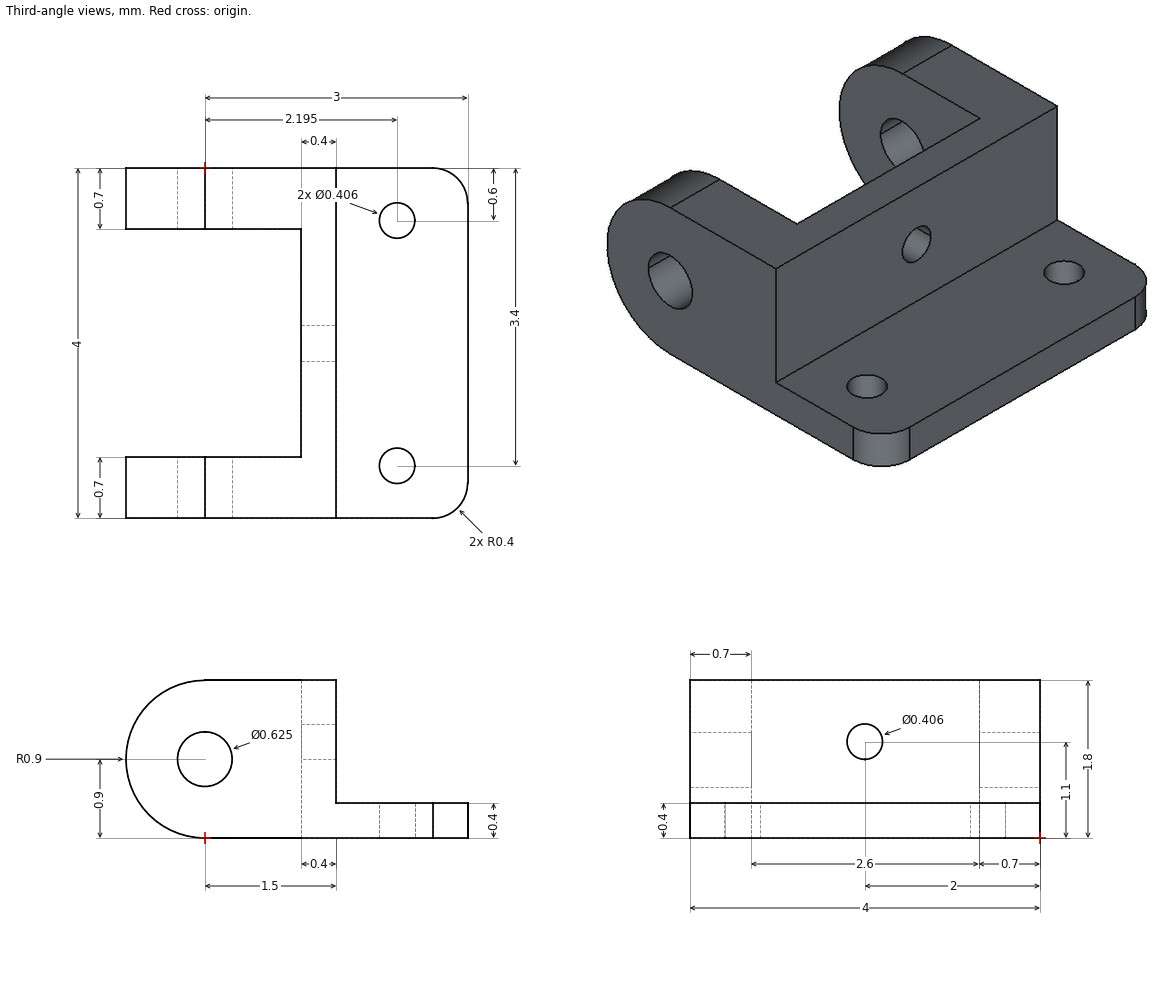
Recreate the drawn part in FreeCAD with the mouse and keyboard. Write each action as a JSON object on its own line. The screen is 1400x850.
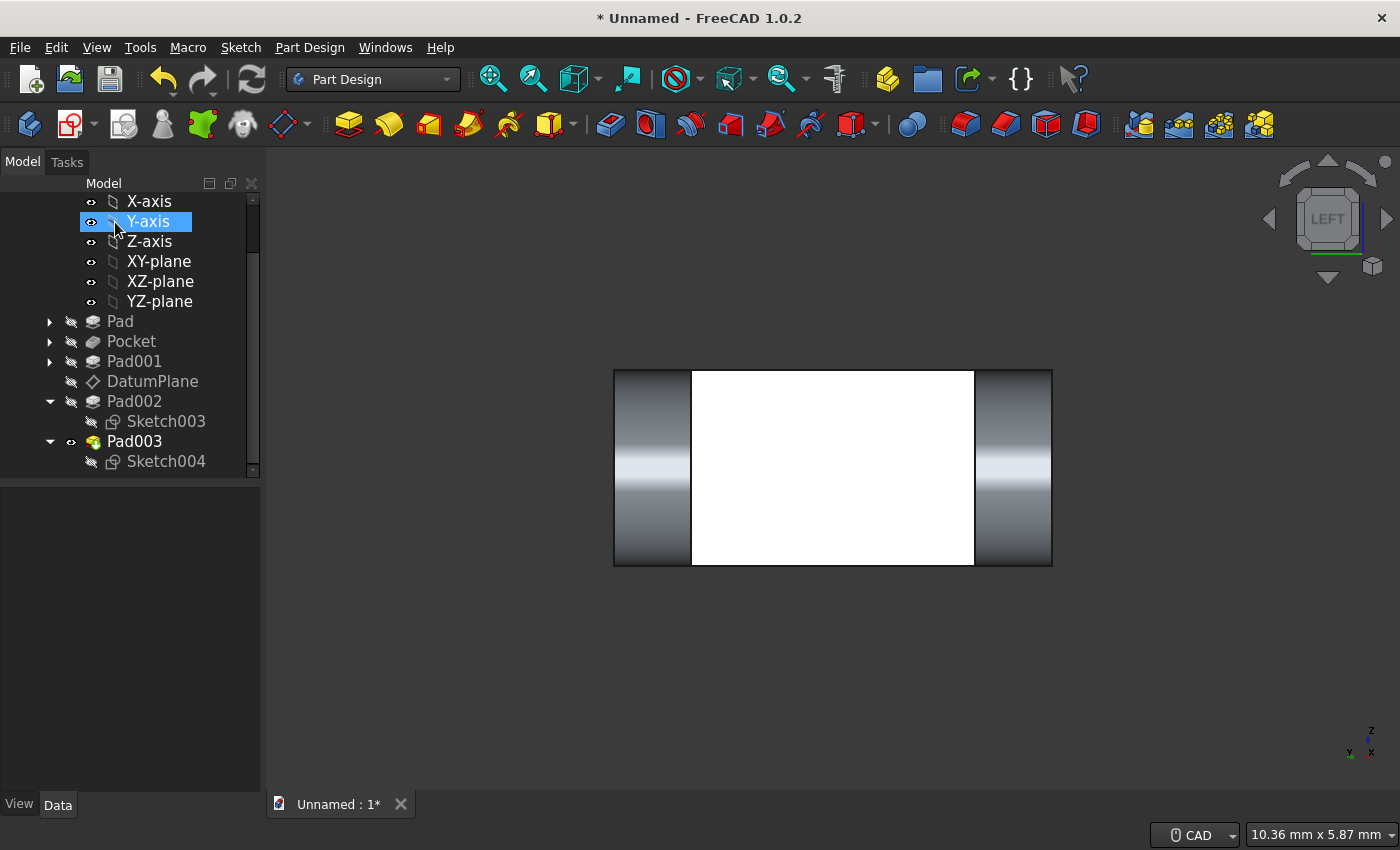
{"action": "key", "text": "0"}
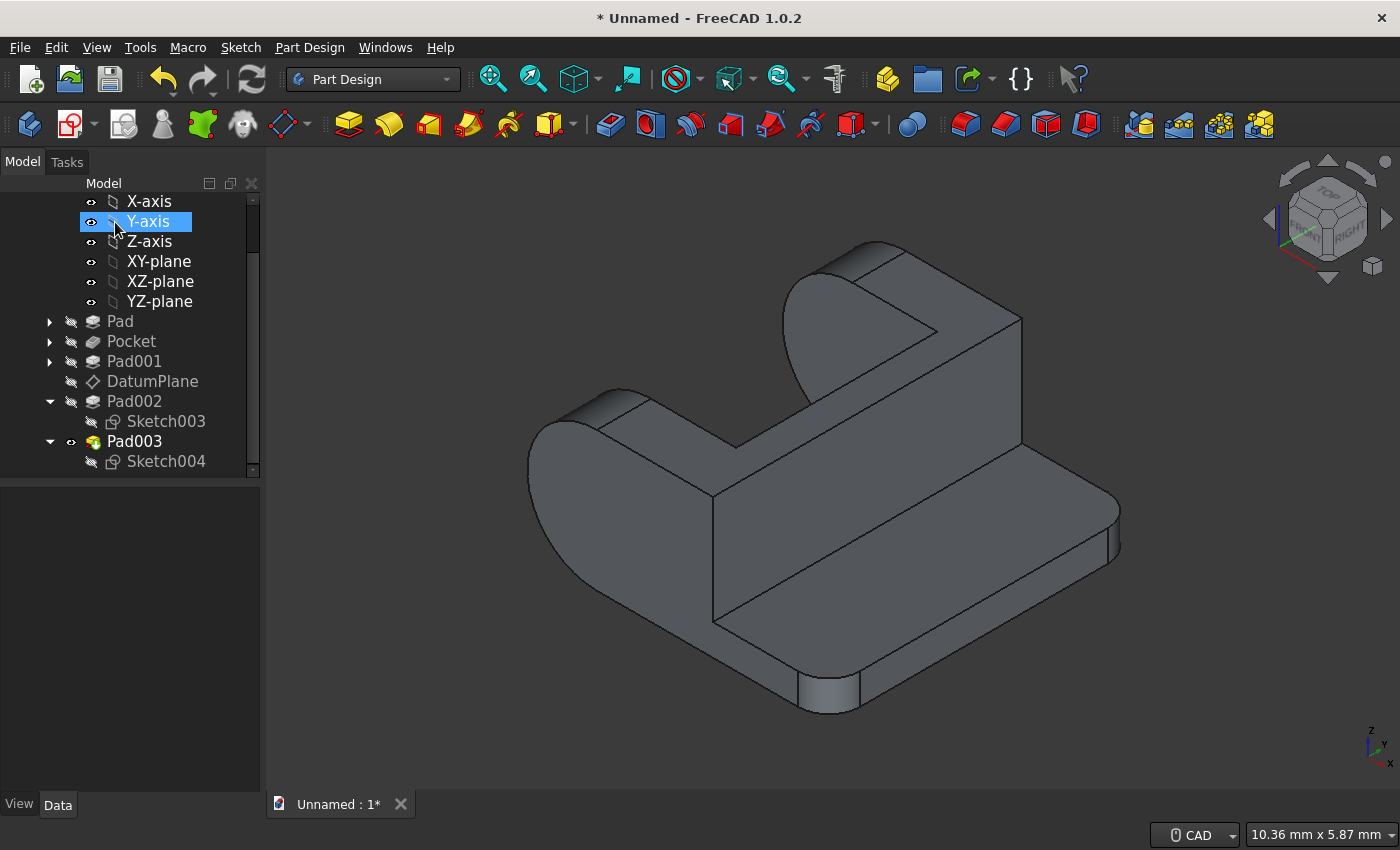
{"action": "left_click", "coordinate": [823, 495]}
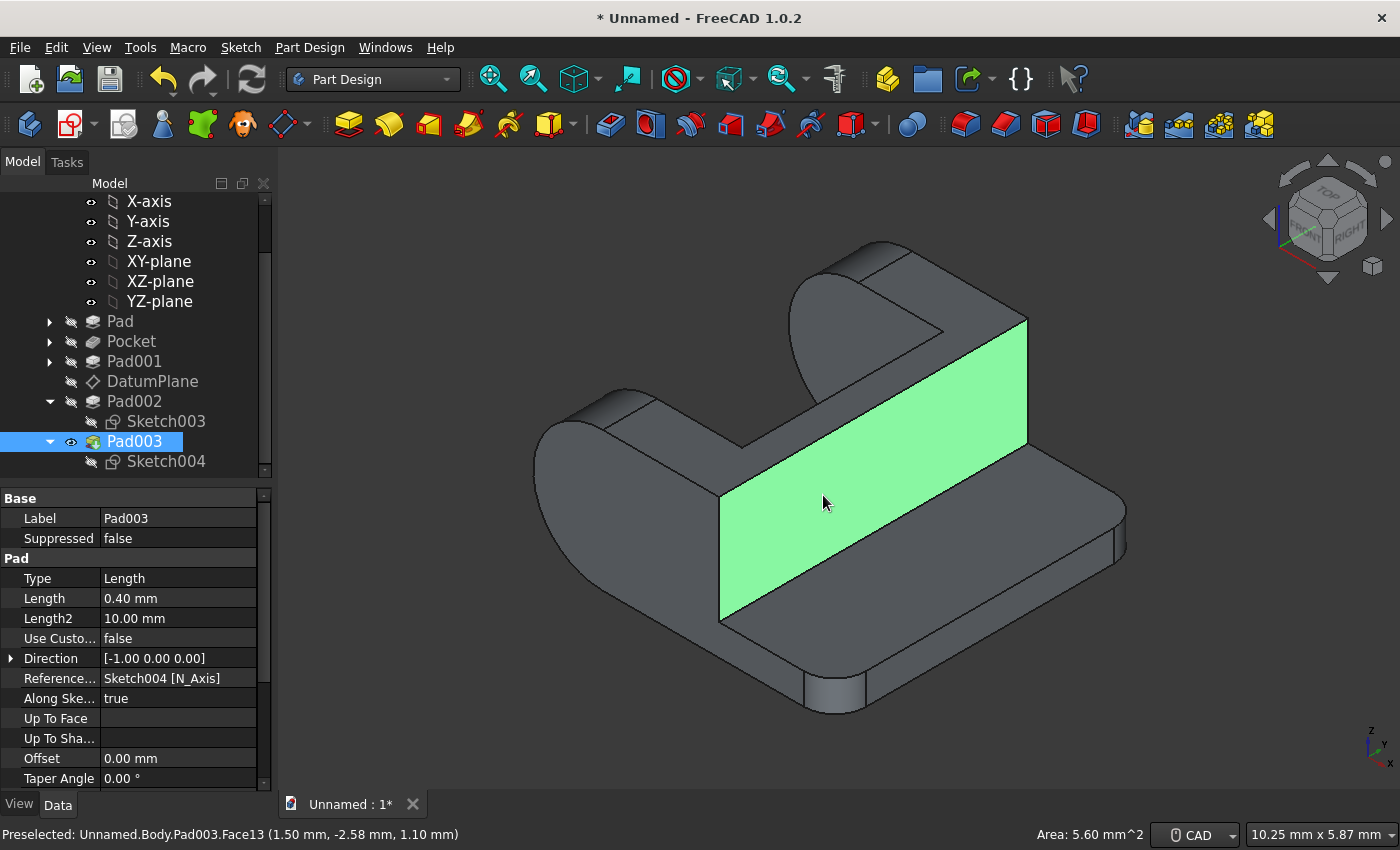
{"action": "left_click", "coordinate": [70, 124]}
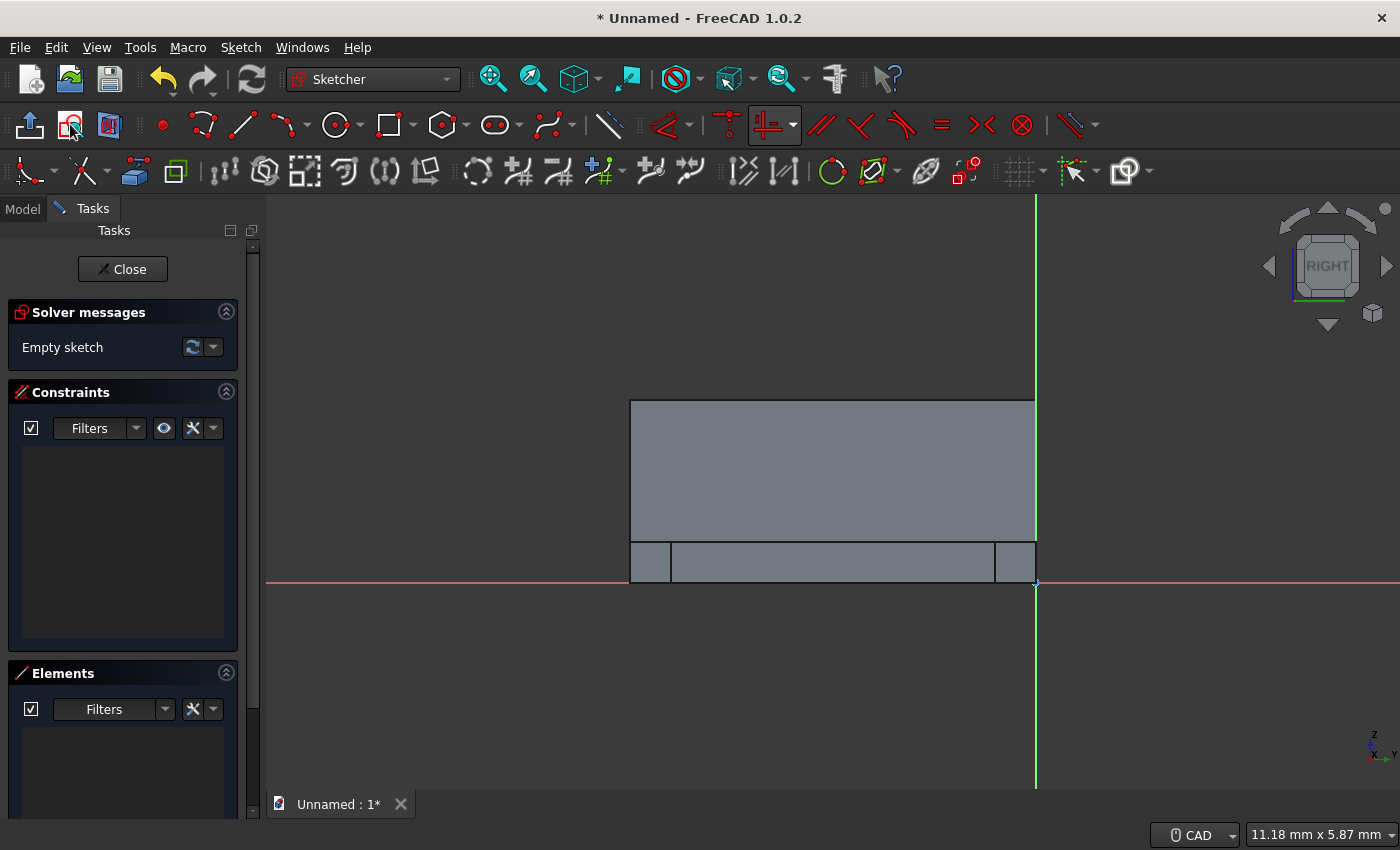
{"action": "key", "text": "q s"}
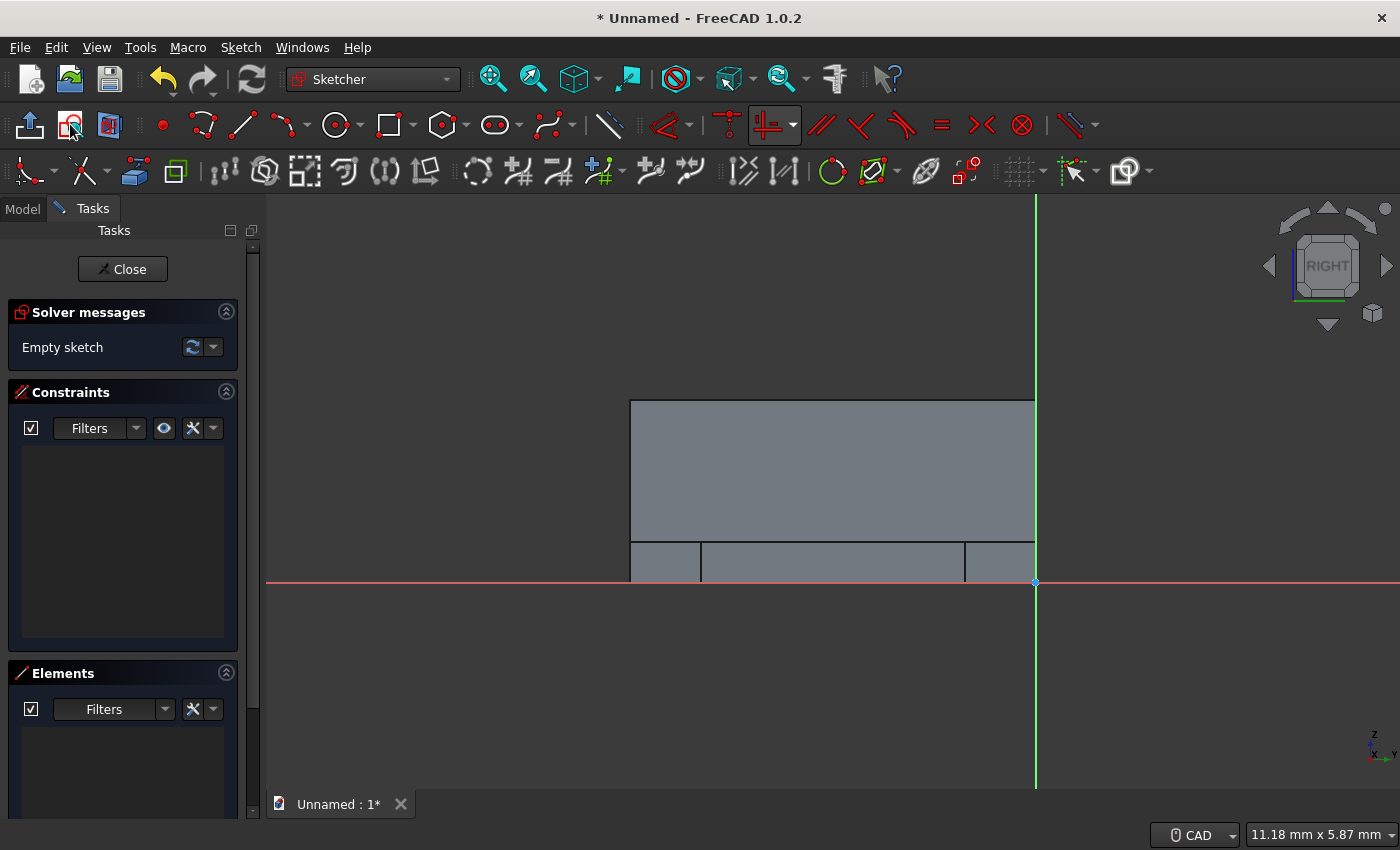
{"action": "scroll", "coordinate": [842, 469], "scroll_direction": "up", "scroll_amount": 11}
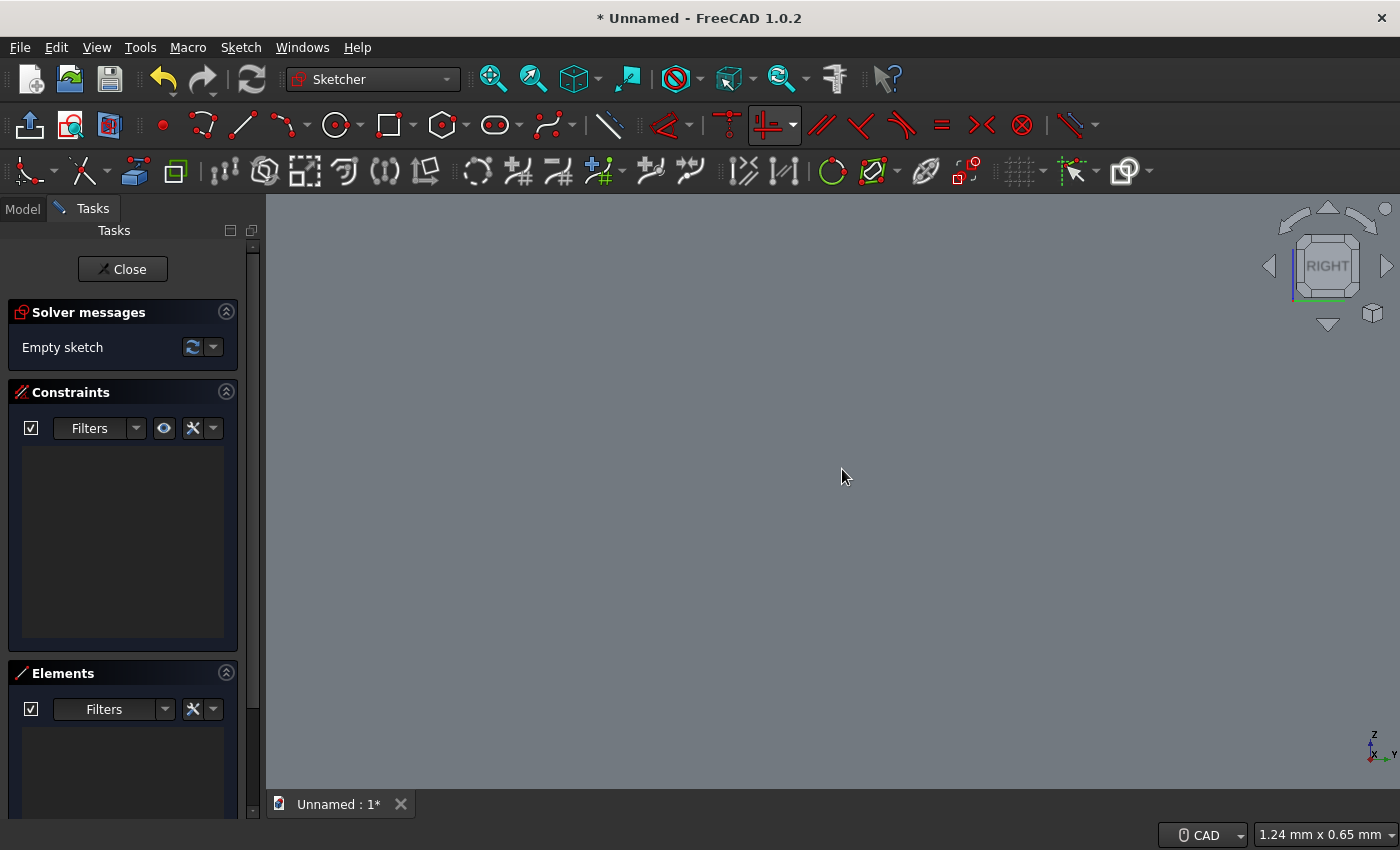
{"action": "key", "text": "g c"}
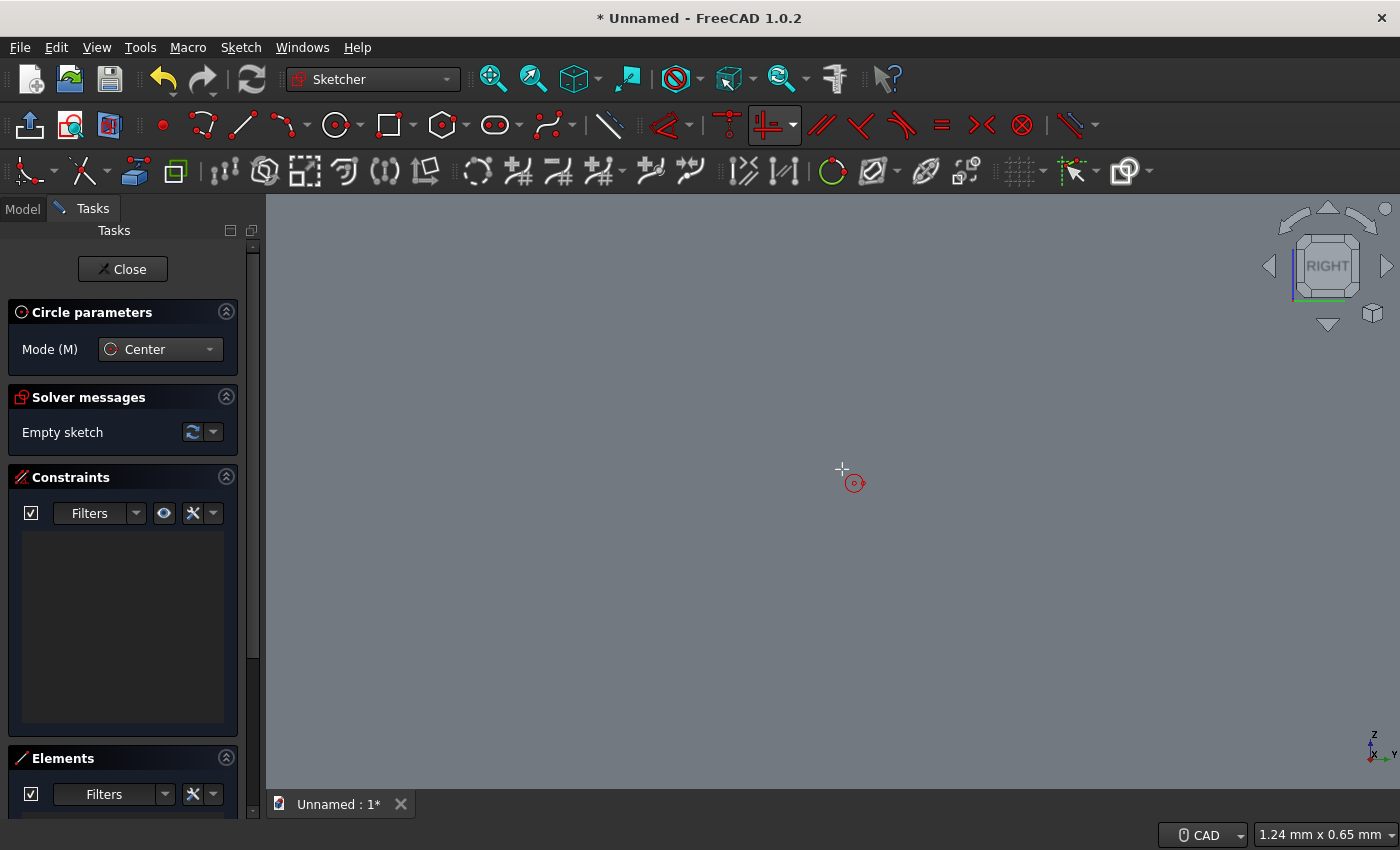
{"action": "left_click", "coordinate": [757, 485]}
{"action": "mouse_move", "coordinate": [888, 354]}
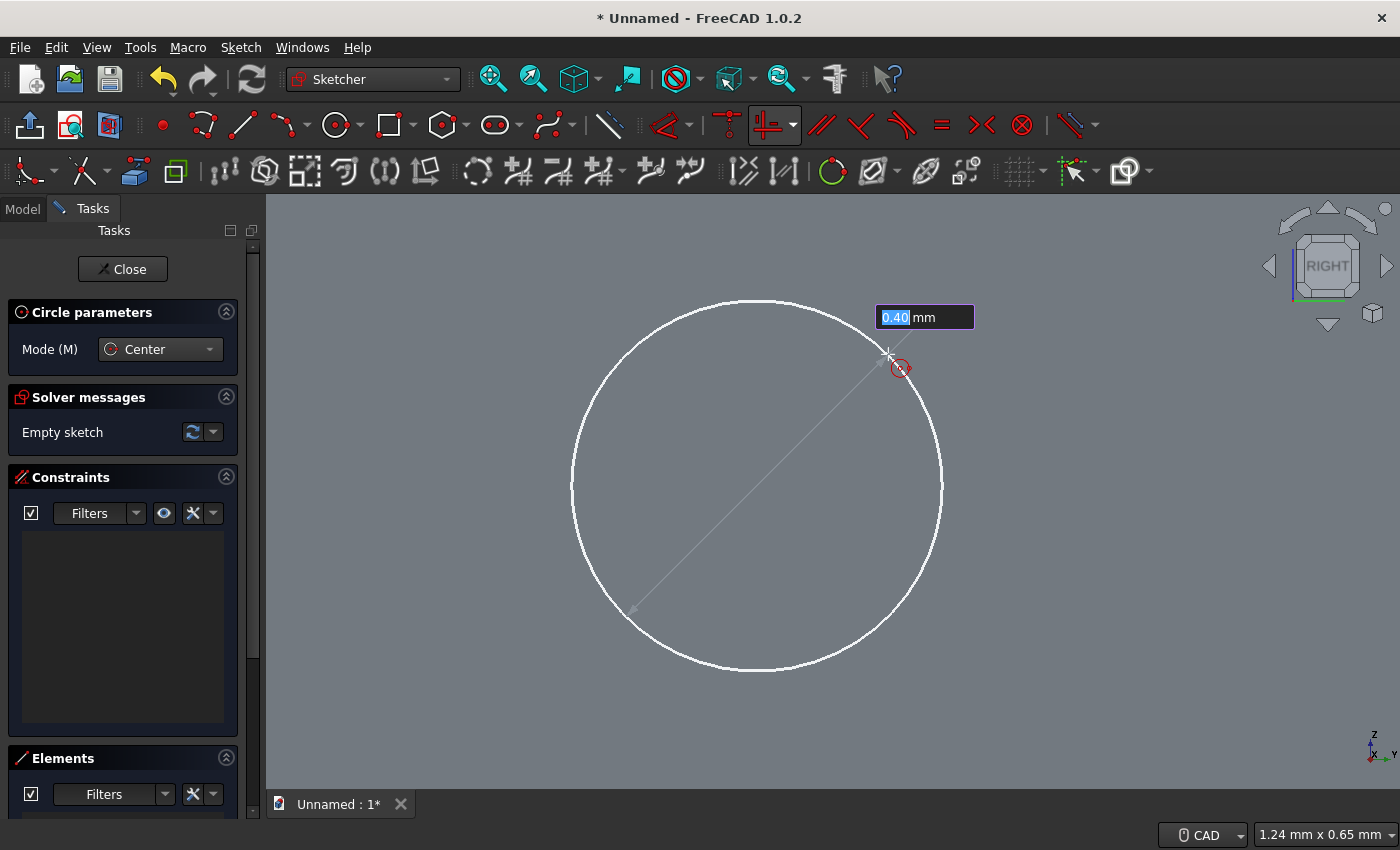
{"action": "type", "text": "0.406"}
{"action": "key", "text": "Return"}
{"action": "key", "text": "Escape"}